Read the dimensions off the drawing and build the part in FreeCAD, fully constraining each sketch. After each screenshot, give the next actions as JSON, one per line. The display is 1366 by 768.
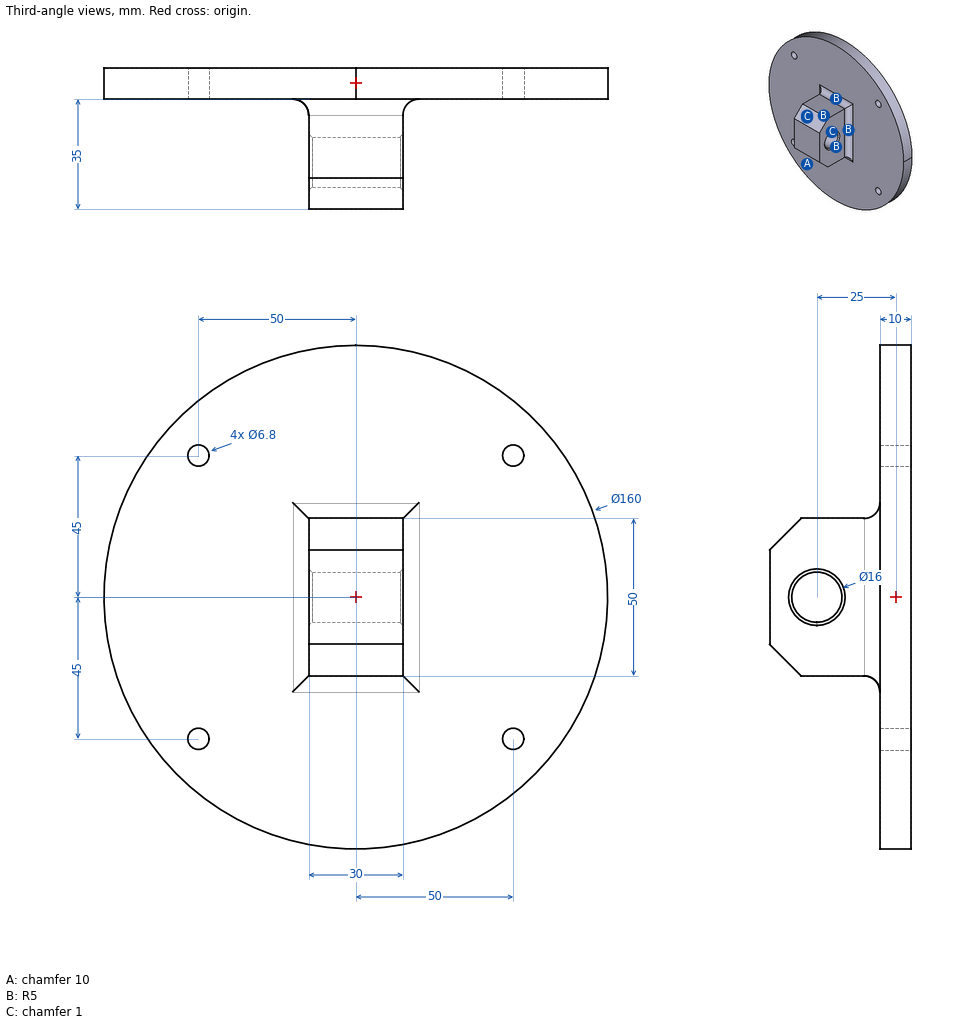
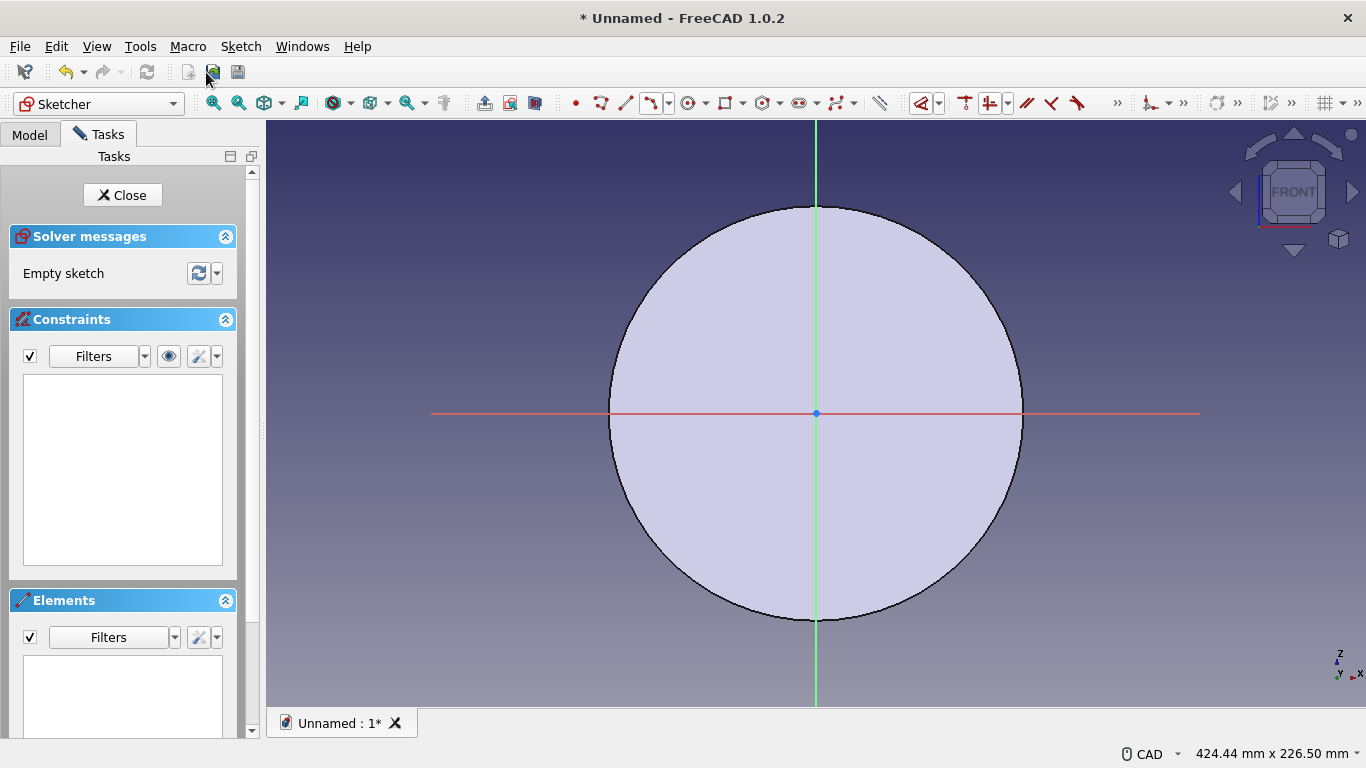
{"action": "scroll", "coordinate": [955, 413], "scroll_direction": "up", "scroll_amount": 2}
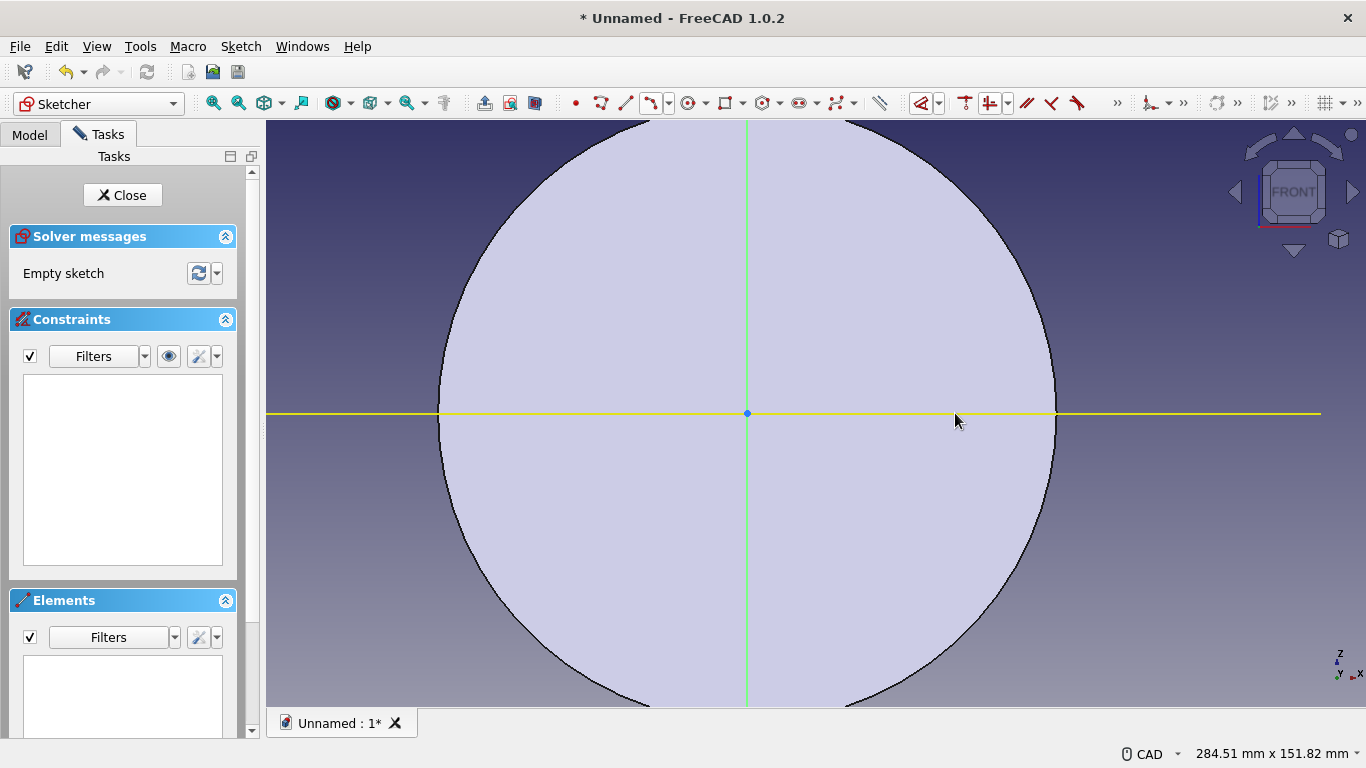
{"action": "left_click", "coordinate": [688, 104]}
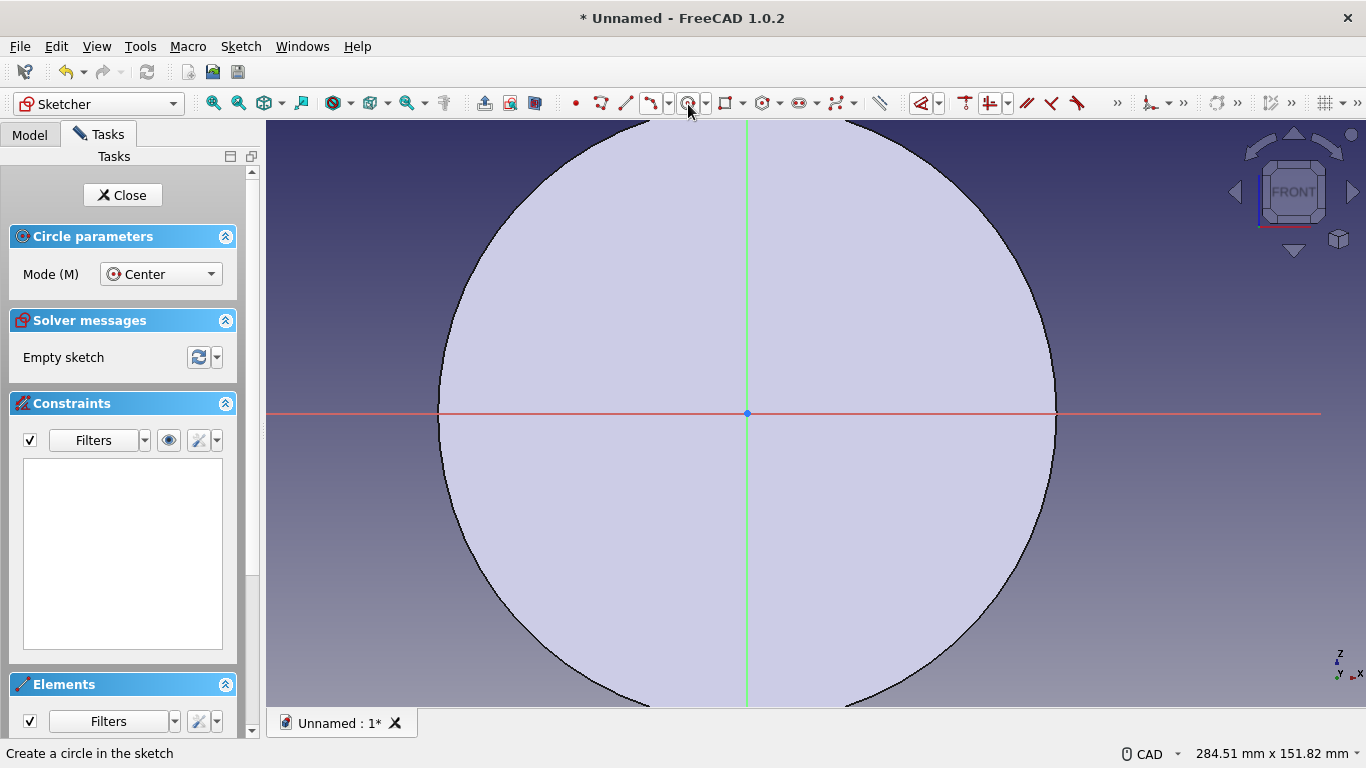
{"action": "scroll", "coordinate": [554, 240], "scroll_direction": "up", "scroll_amount": 3}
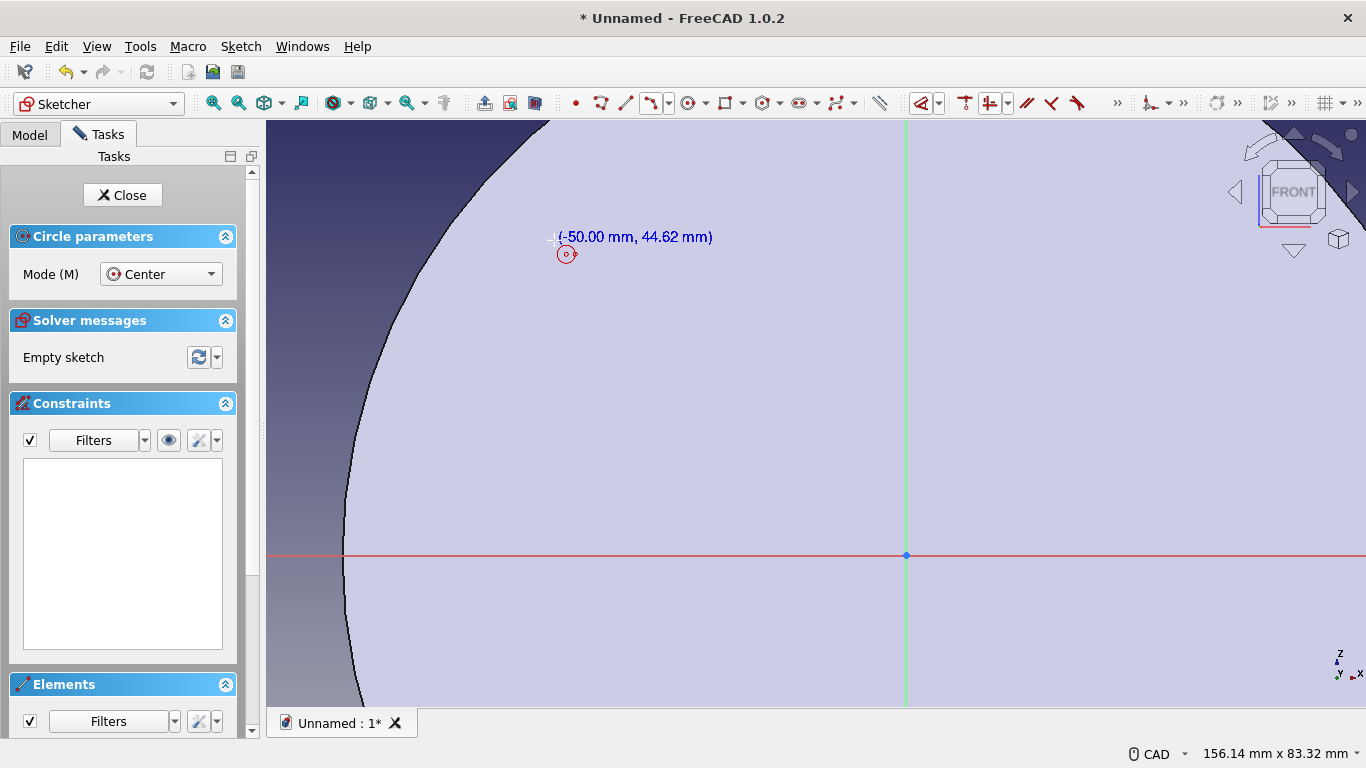
{"action": "left_click", "coordinate": [554, 239]}
{"action": "left_click", "coordinate": [571, 222]}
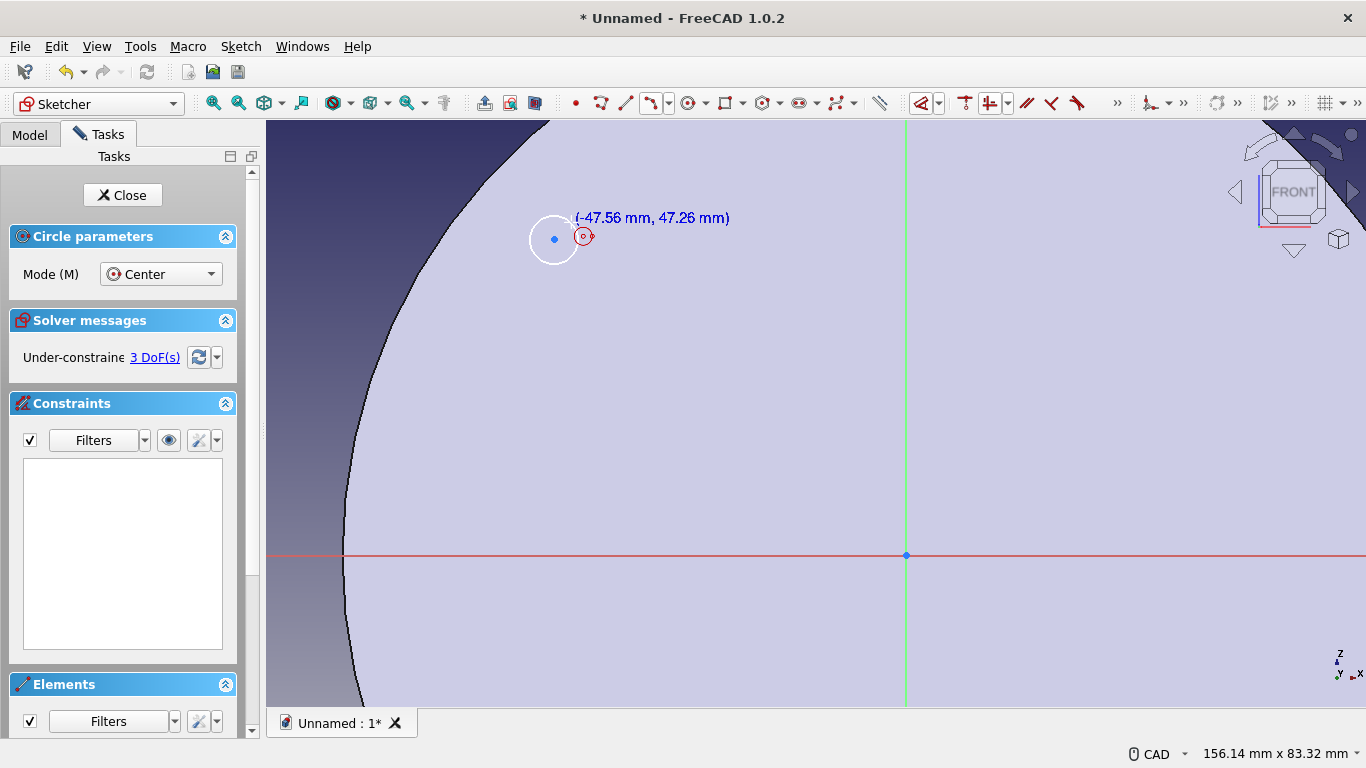
{"action": "scroll", "coordinate": [555, 240], "scroll_direction": "down", "scroll_amount": 3}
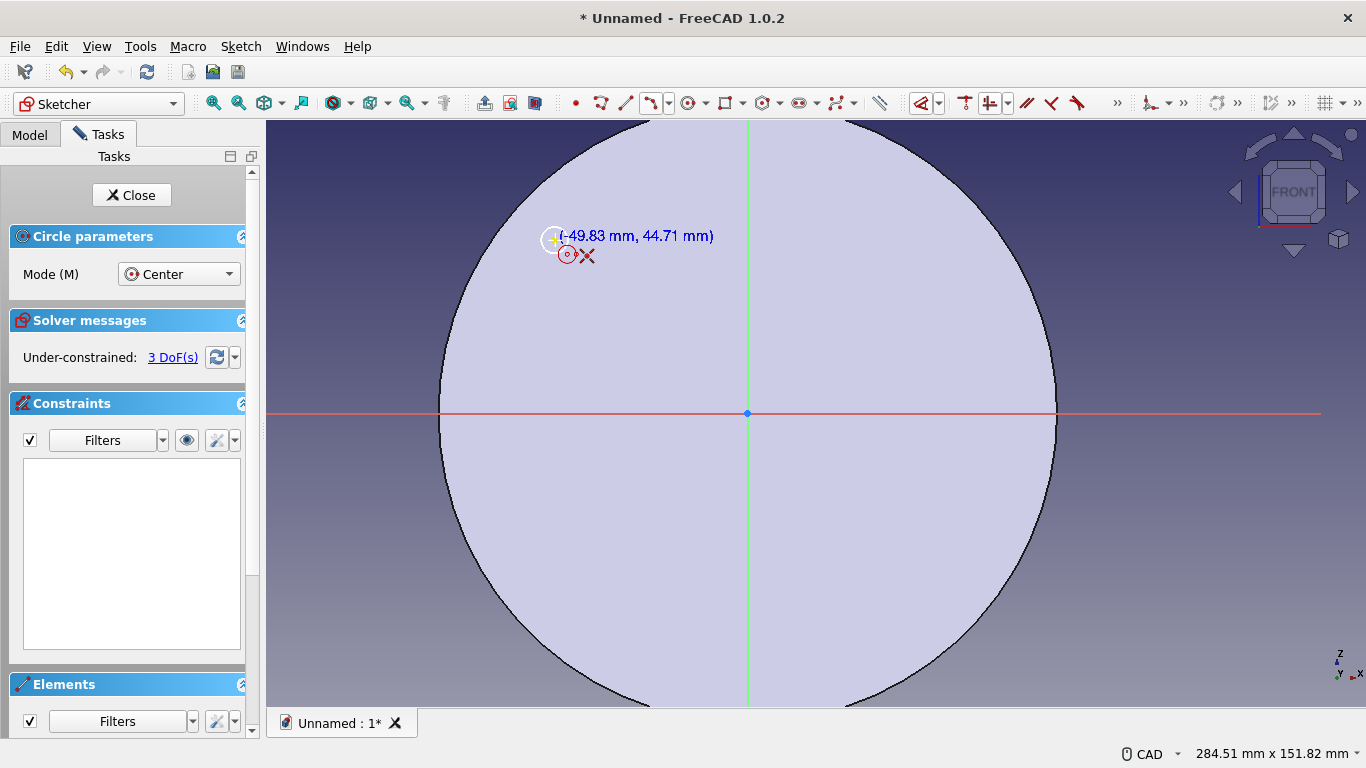
{"action": "scroll", "coordinate": [554, 587], "scroll_direction": "up", "scroll_amount": 3}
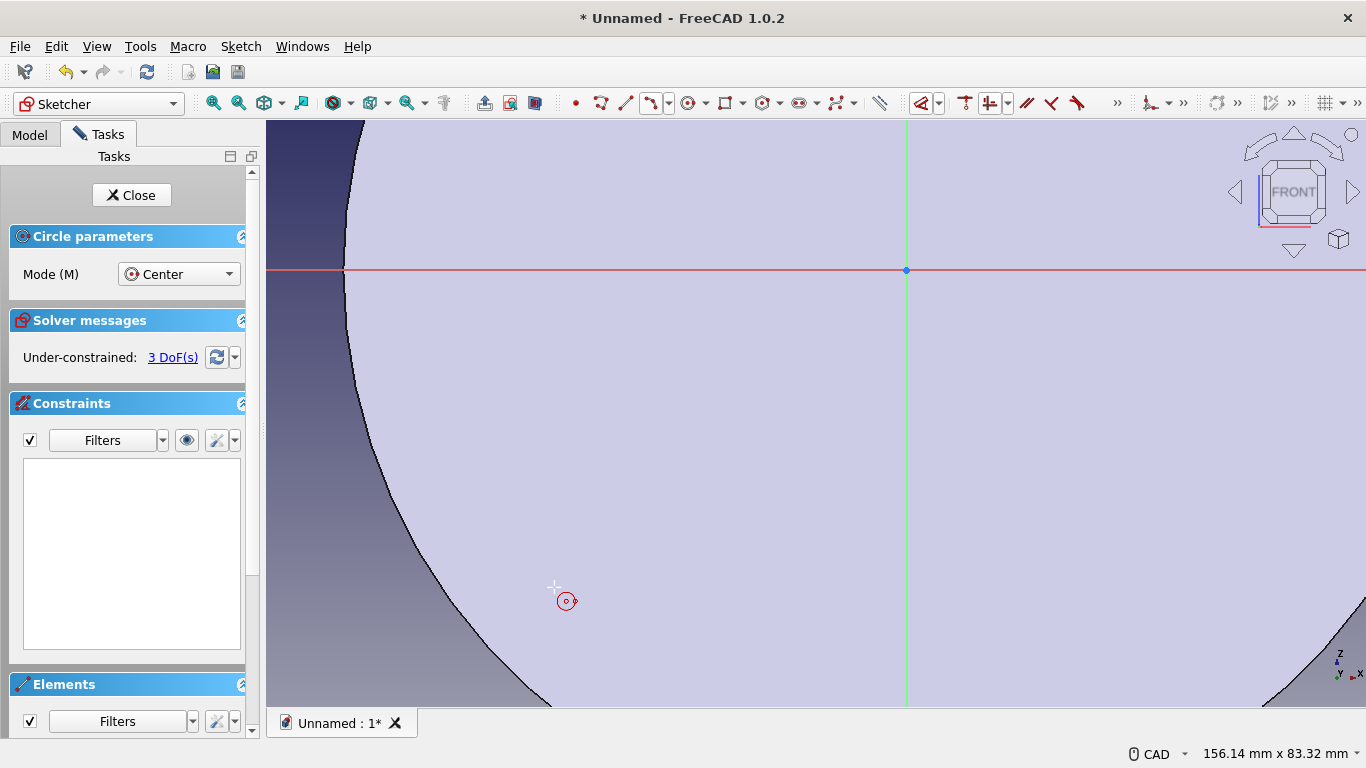
{"action": "left_click", "coordinate": [555, 587]}
{"action": "left_click", "coordinate": [572, 570]}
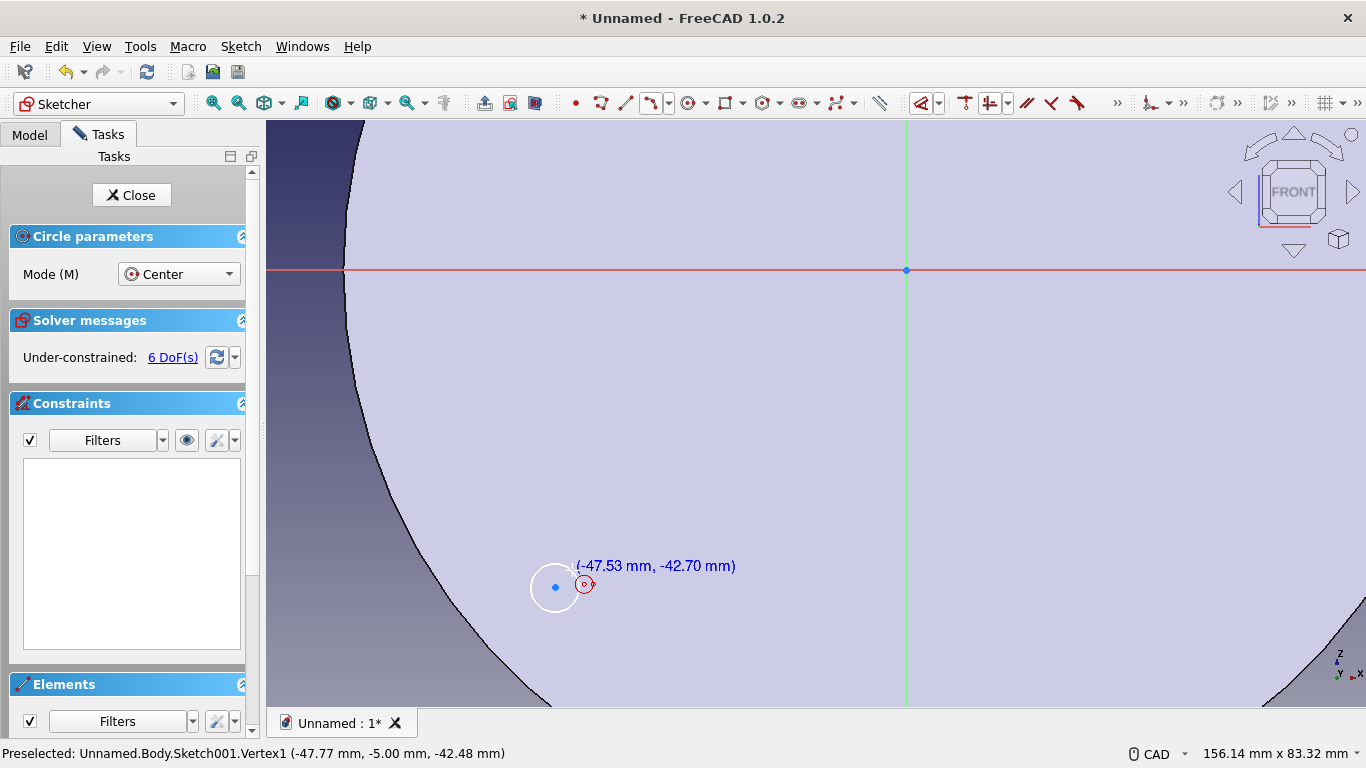
{"action": "scroll", "coordinate": [554, 588], "scroll_direction": "down", "scroll_amount": 3}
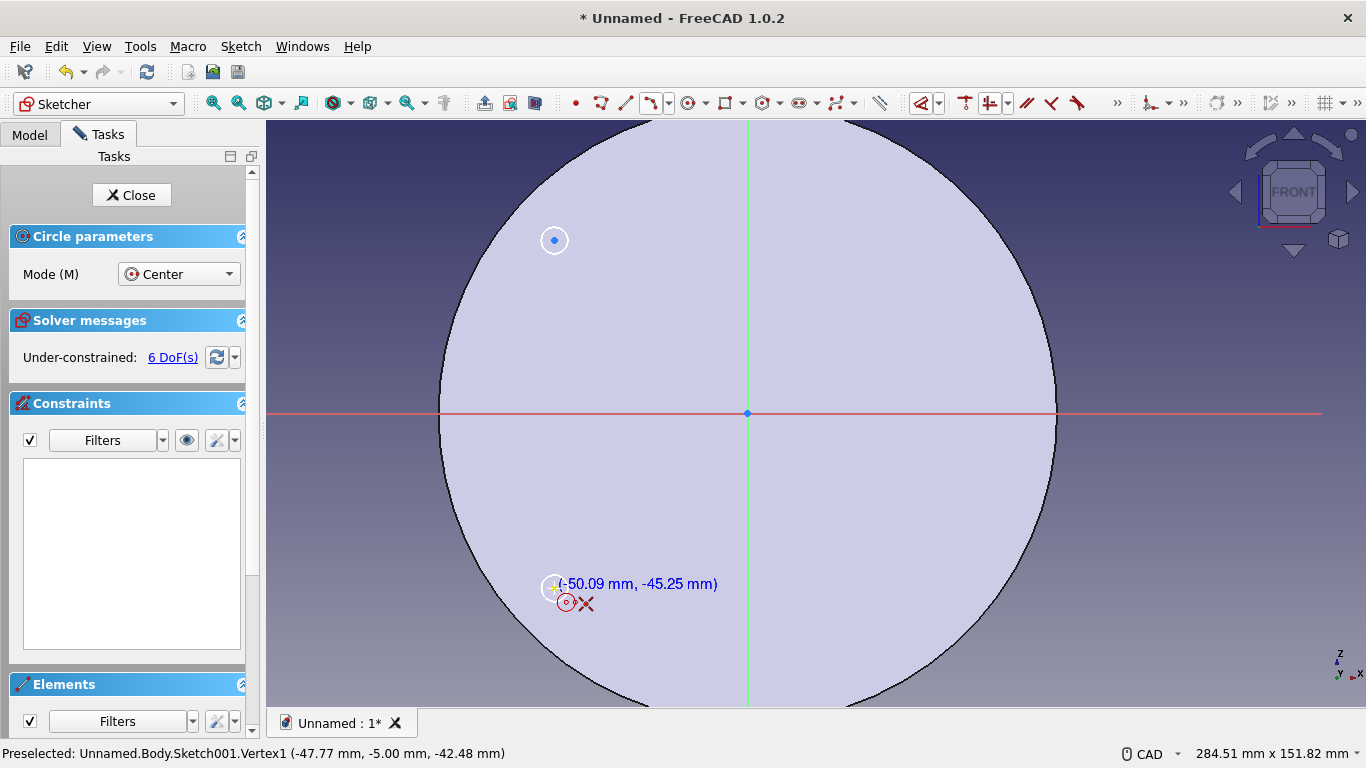
{"action": "scroll", "coordinate": [941, 588], "scroll_direction": "up", "scroll_amount": 3}